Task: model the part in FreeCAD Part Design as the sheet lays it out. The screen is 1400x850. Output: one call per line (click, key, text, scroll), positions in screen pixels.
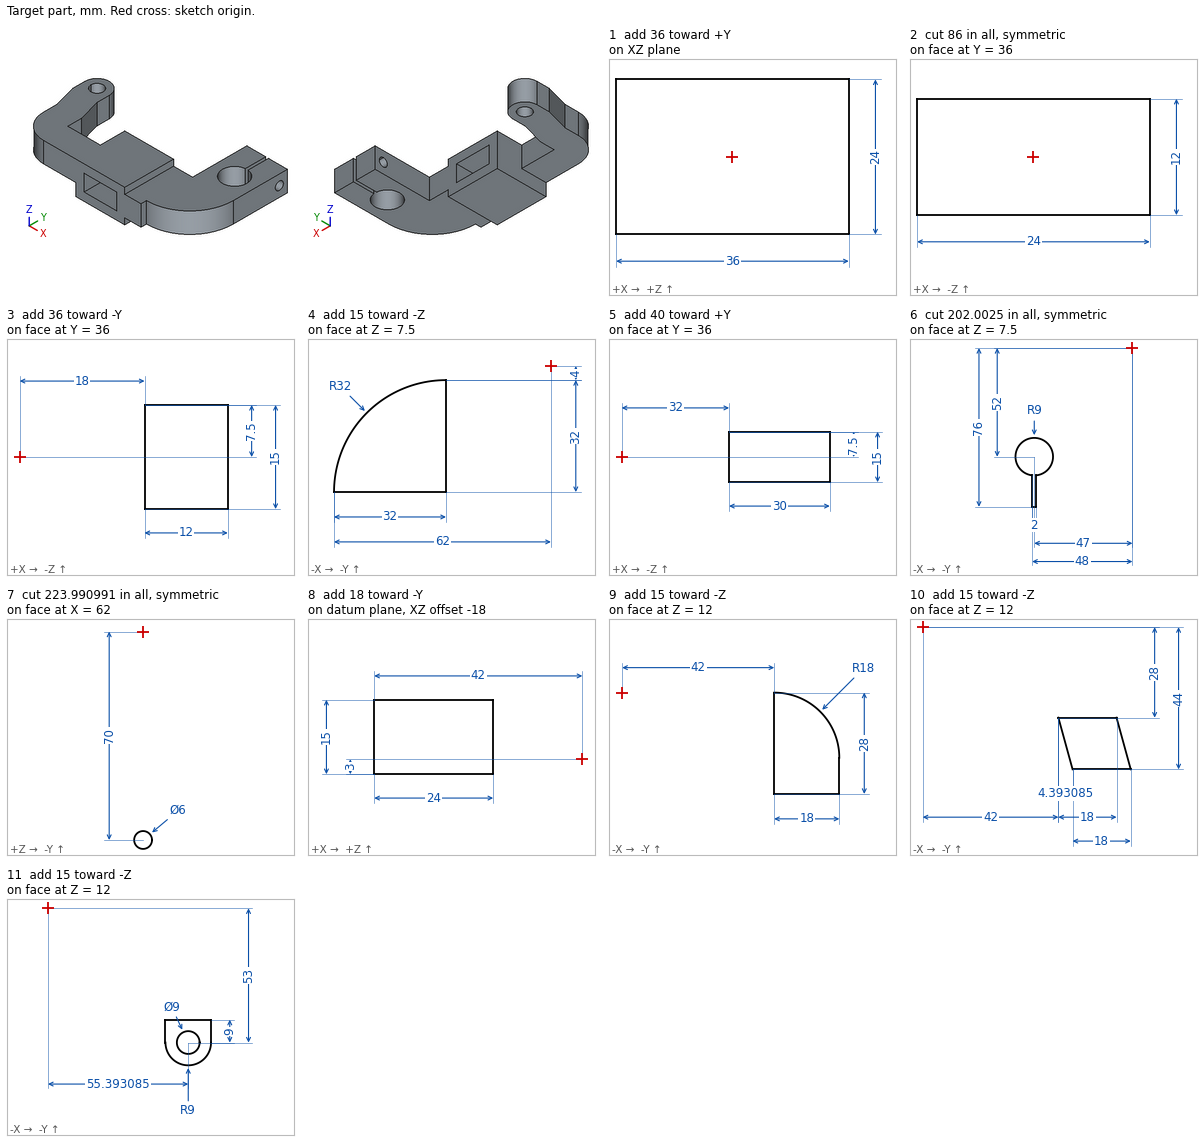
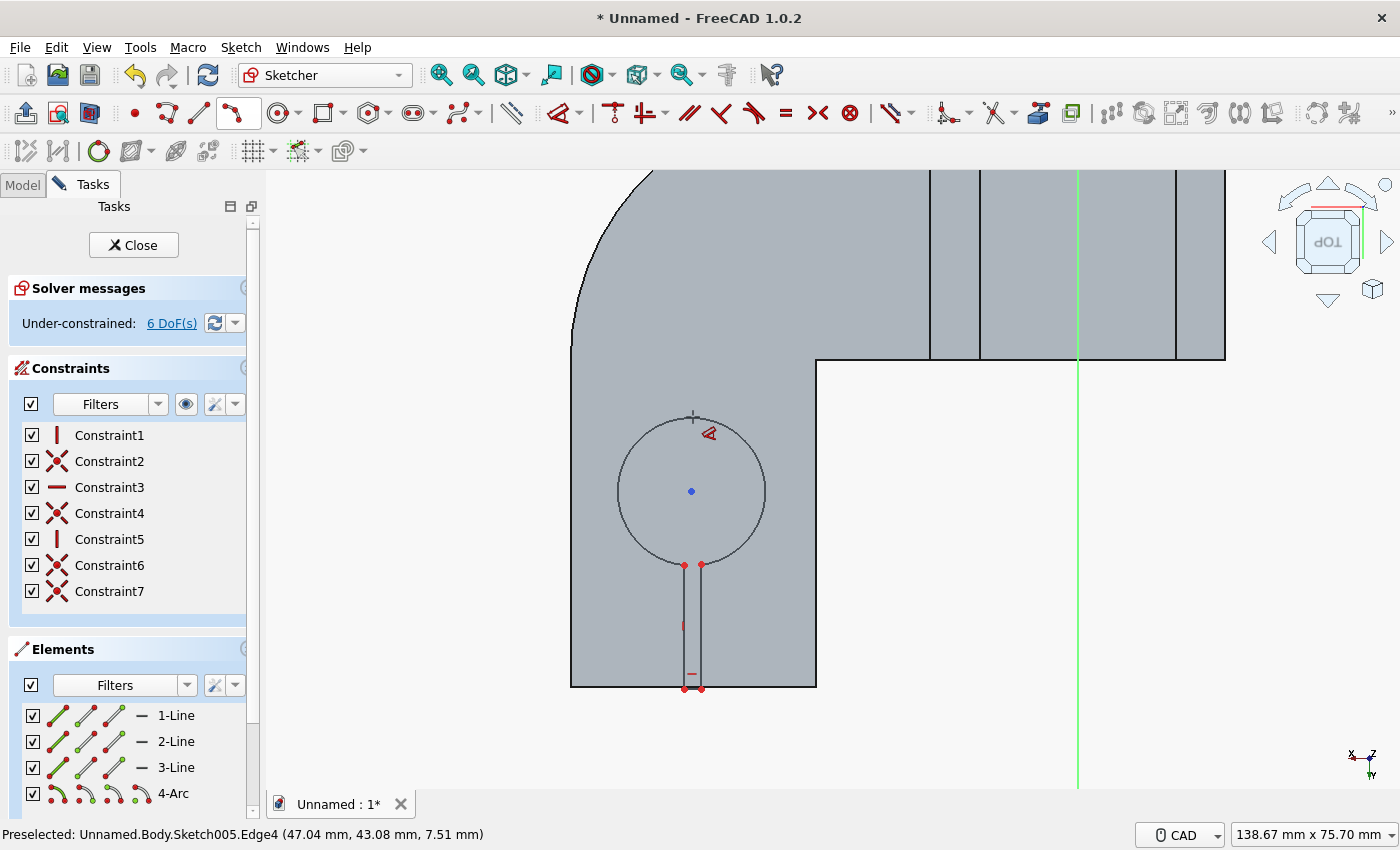
click(760, 465)
click(790, 453)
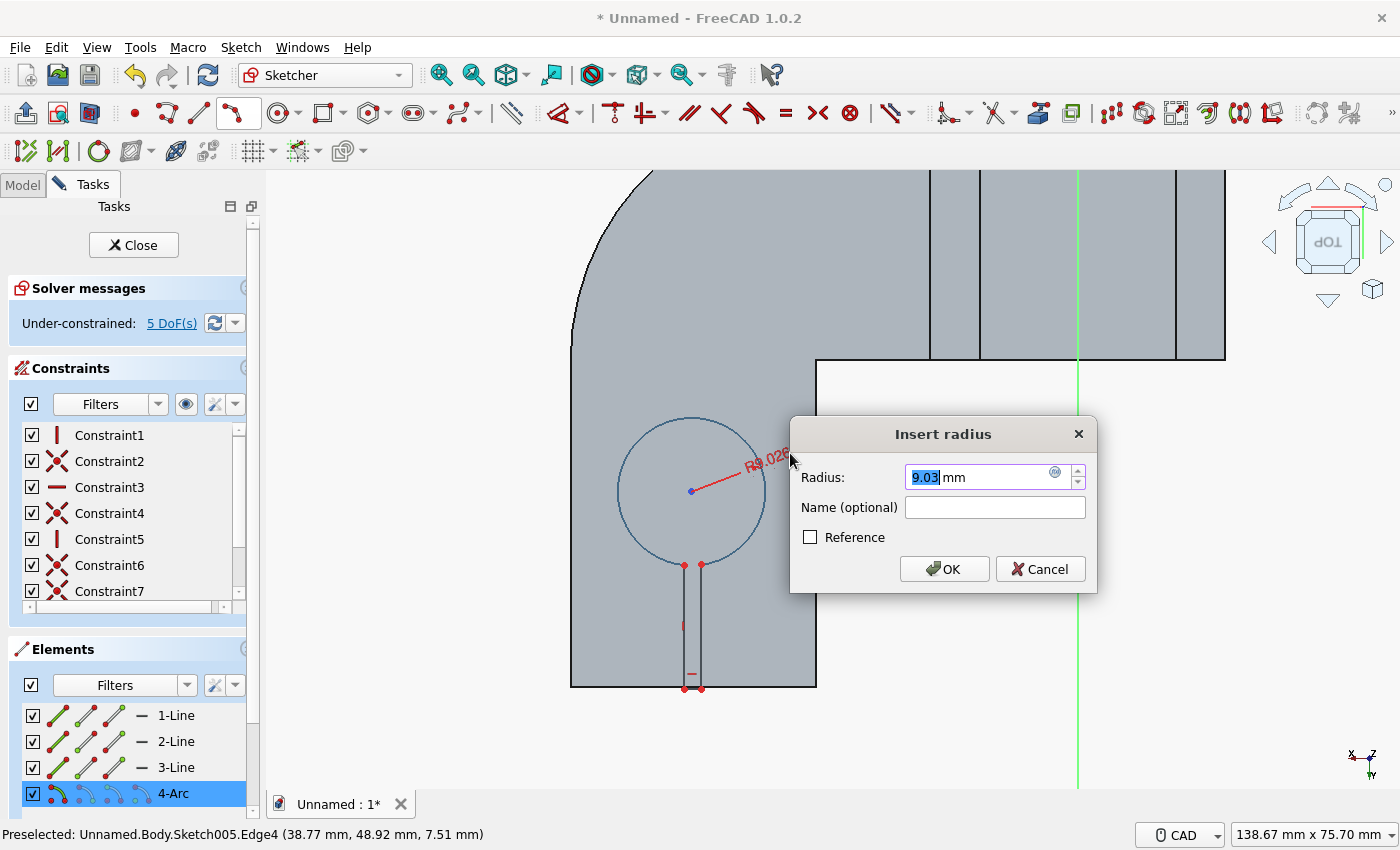
text(9)
key(Return)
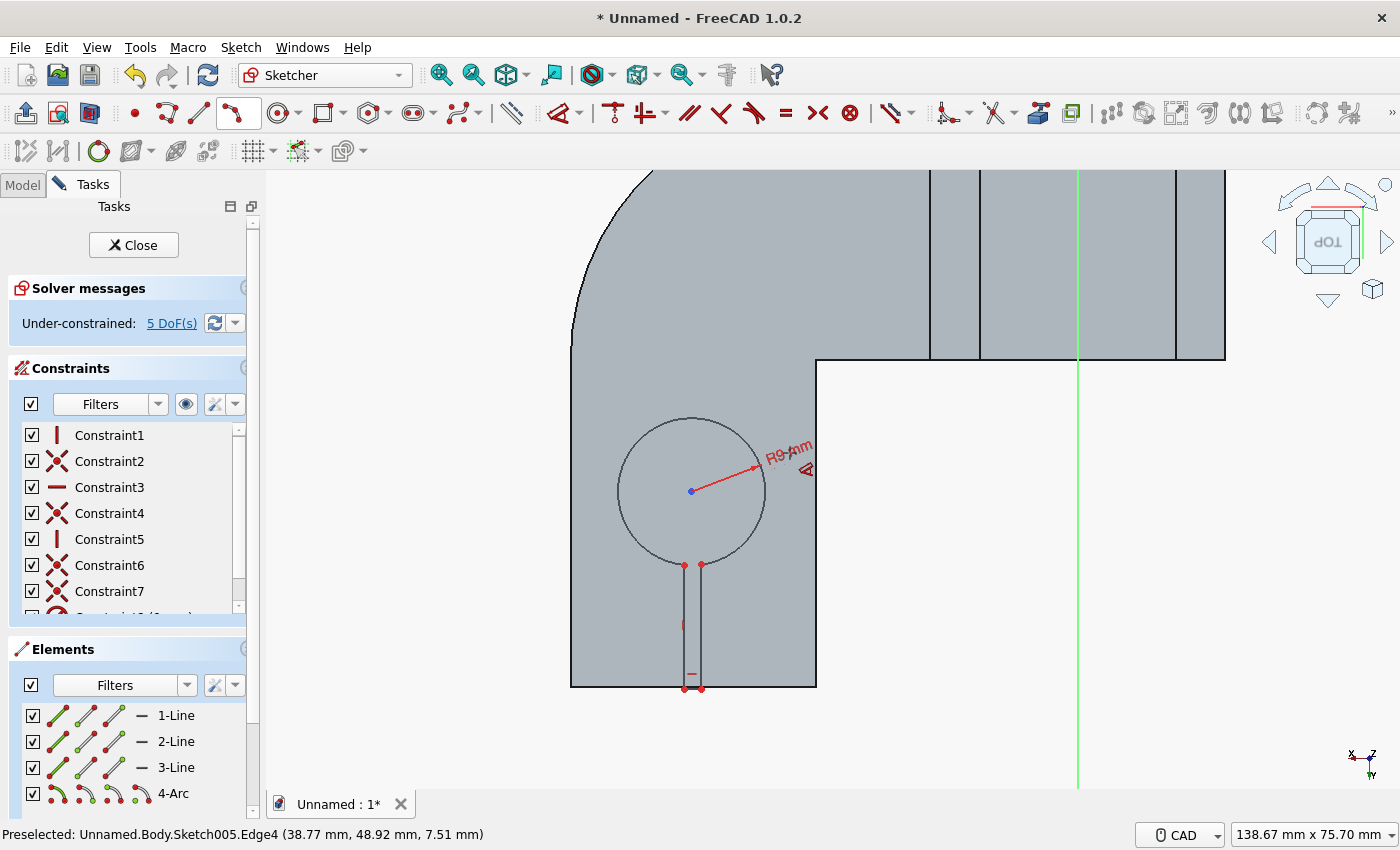
scroll(693, 689, up, 5)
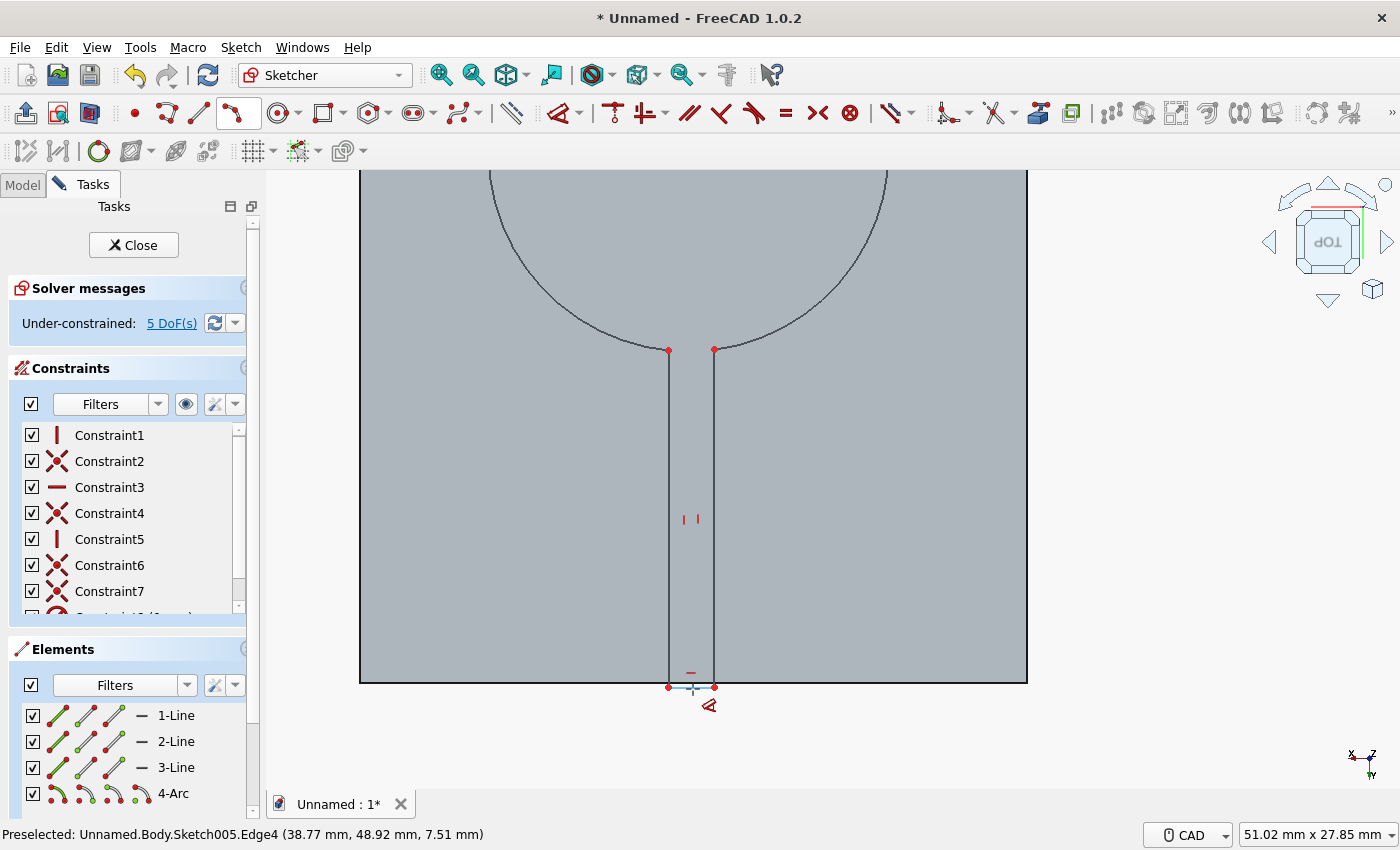
click(692, 688)
click(692, 722)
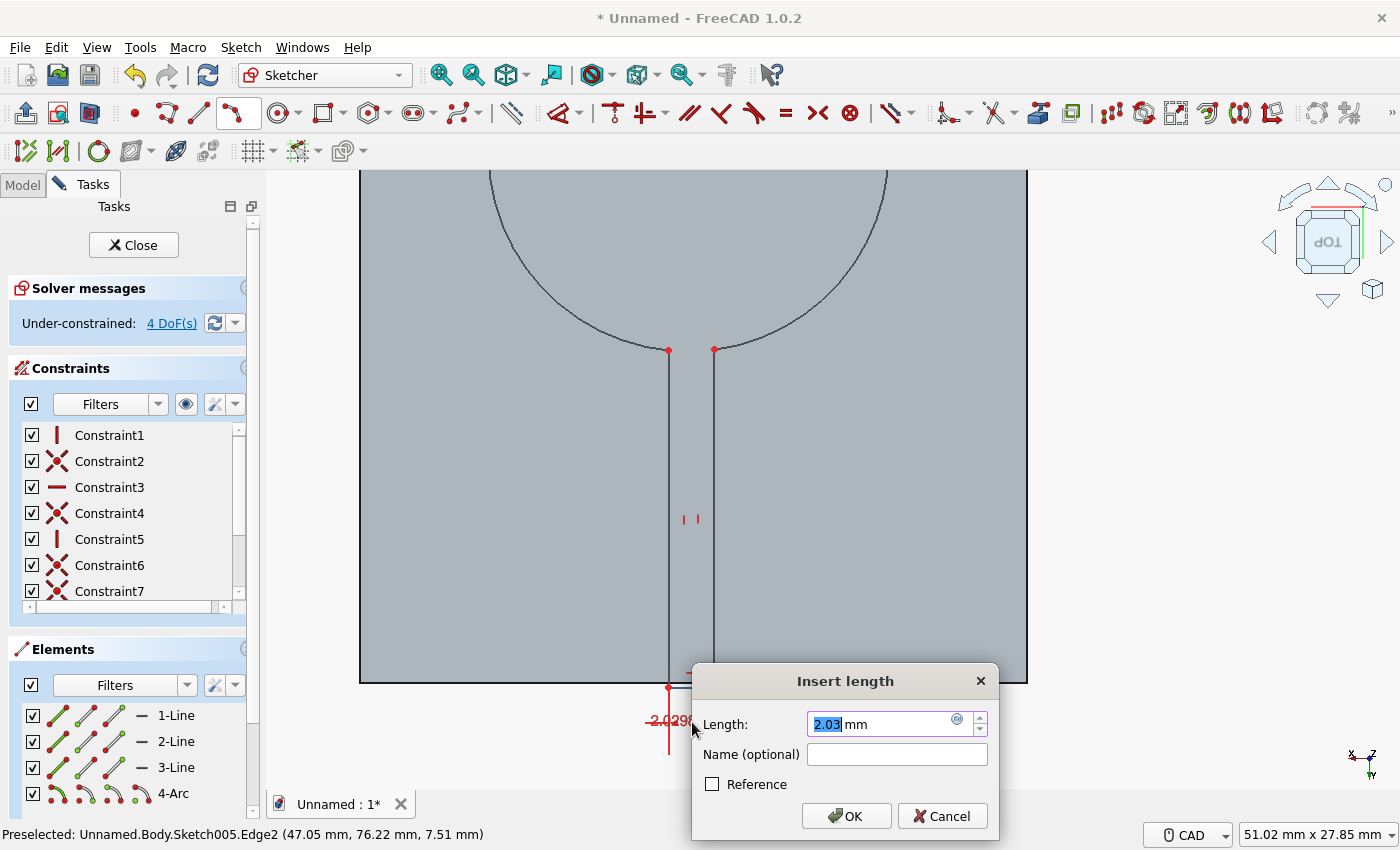
text(2)
key(Return)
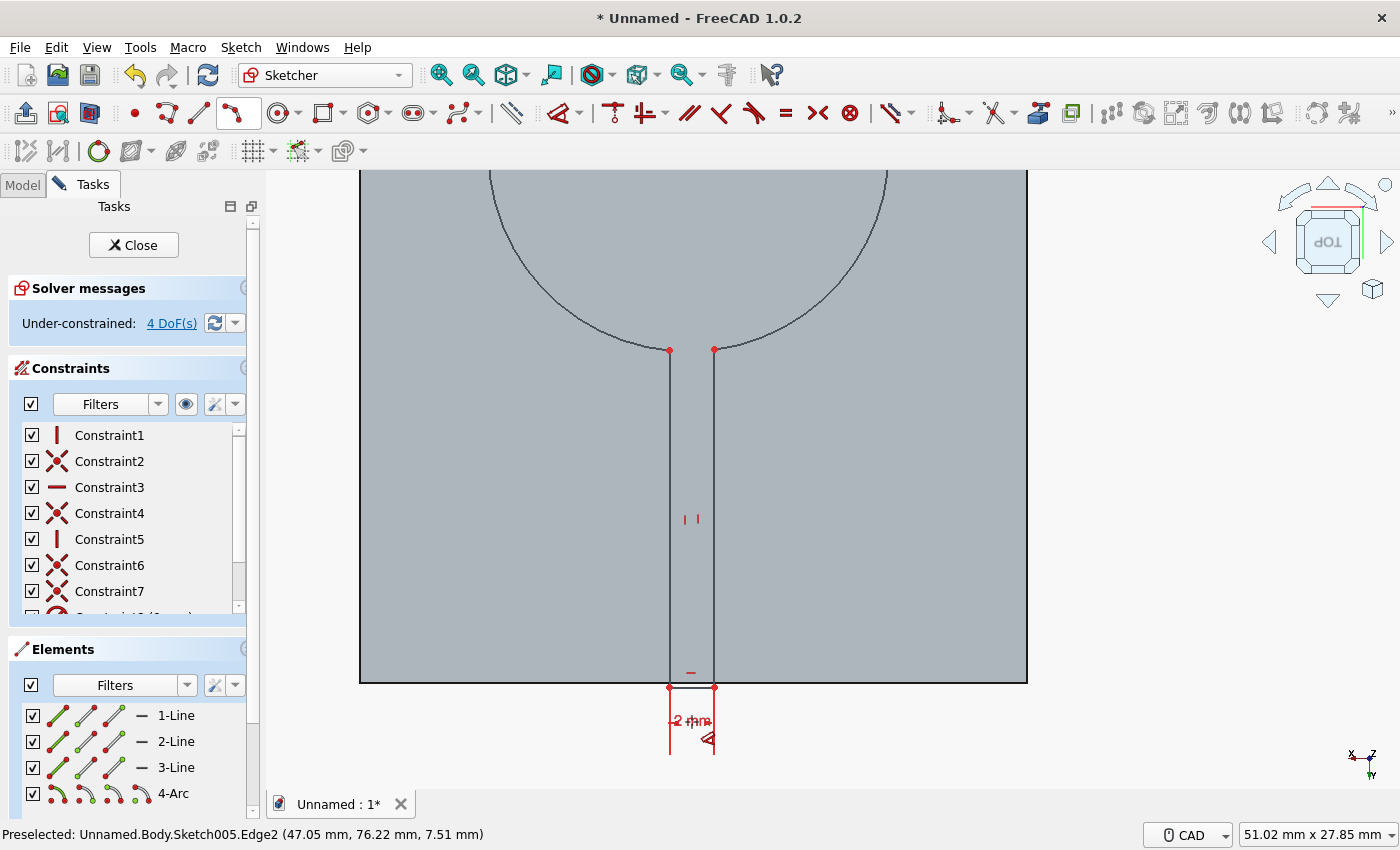
scroll(621, 689, down, 7)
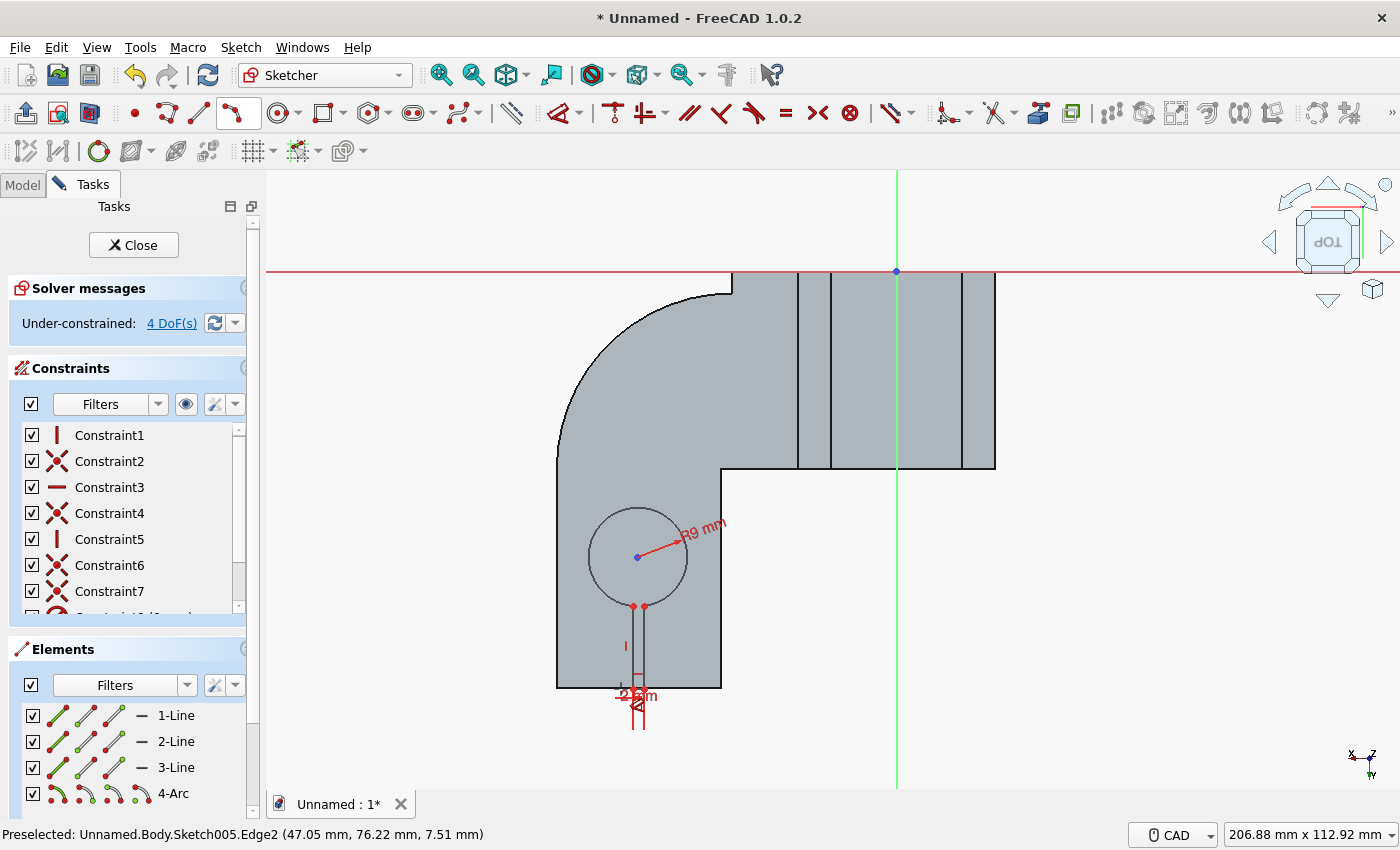
click(633, 606)
click(765, 238)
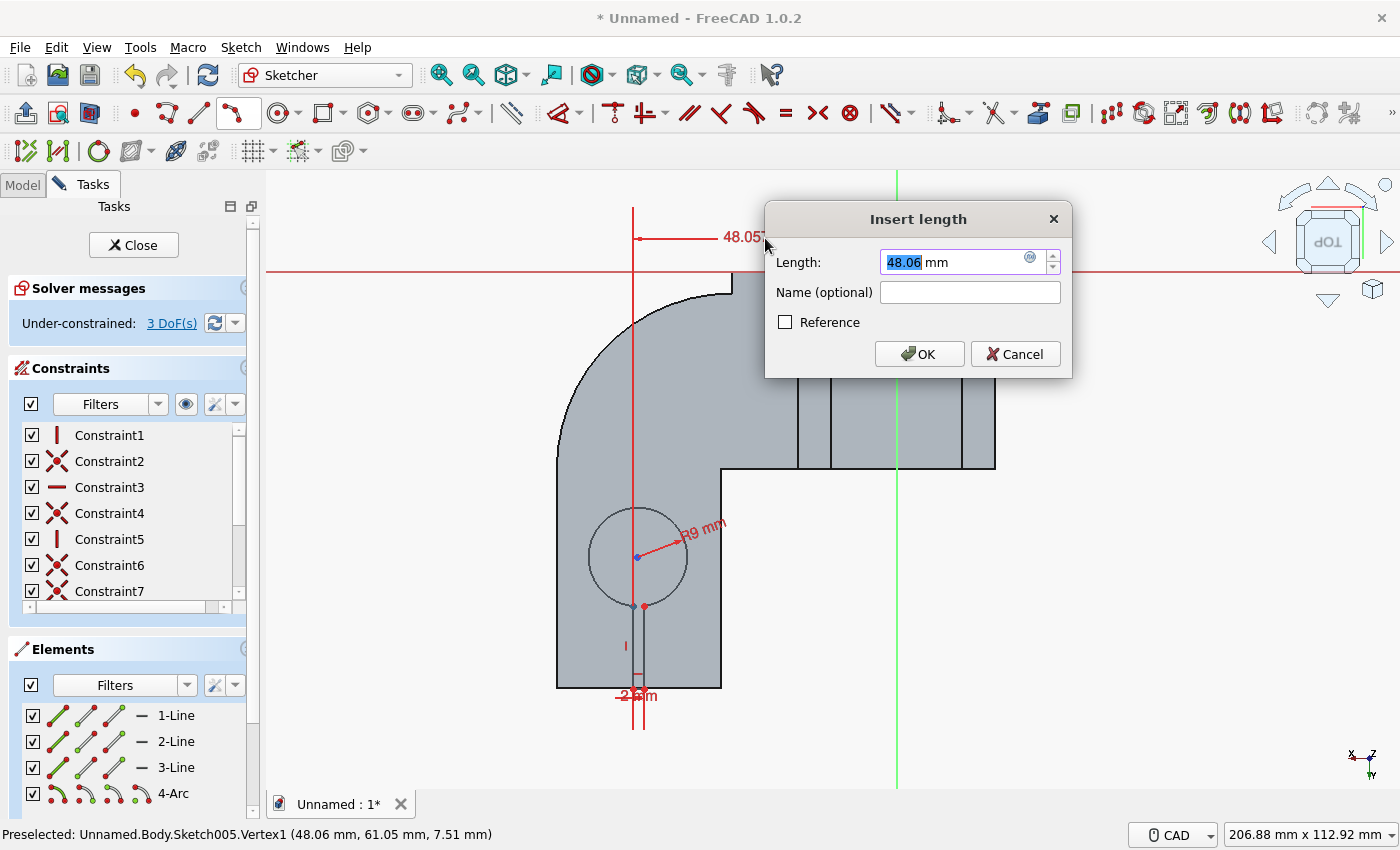
text(48)
key(Return)